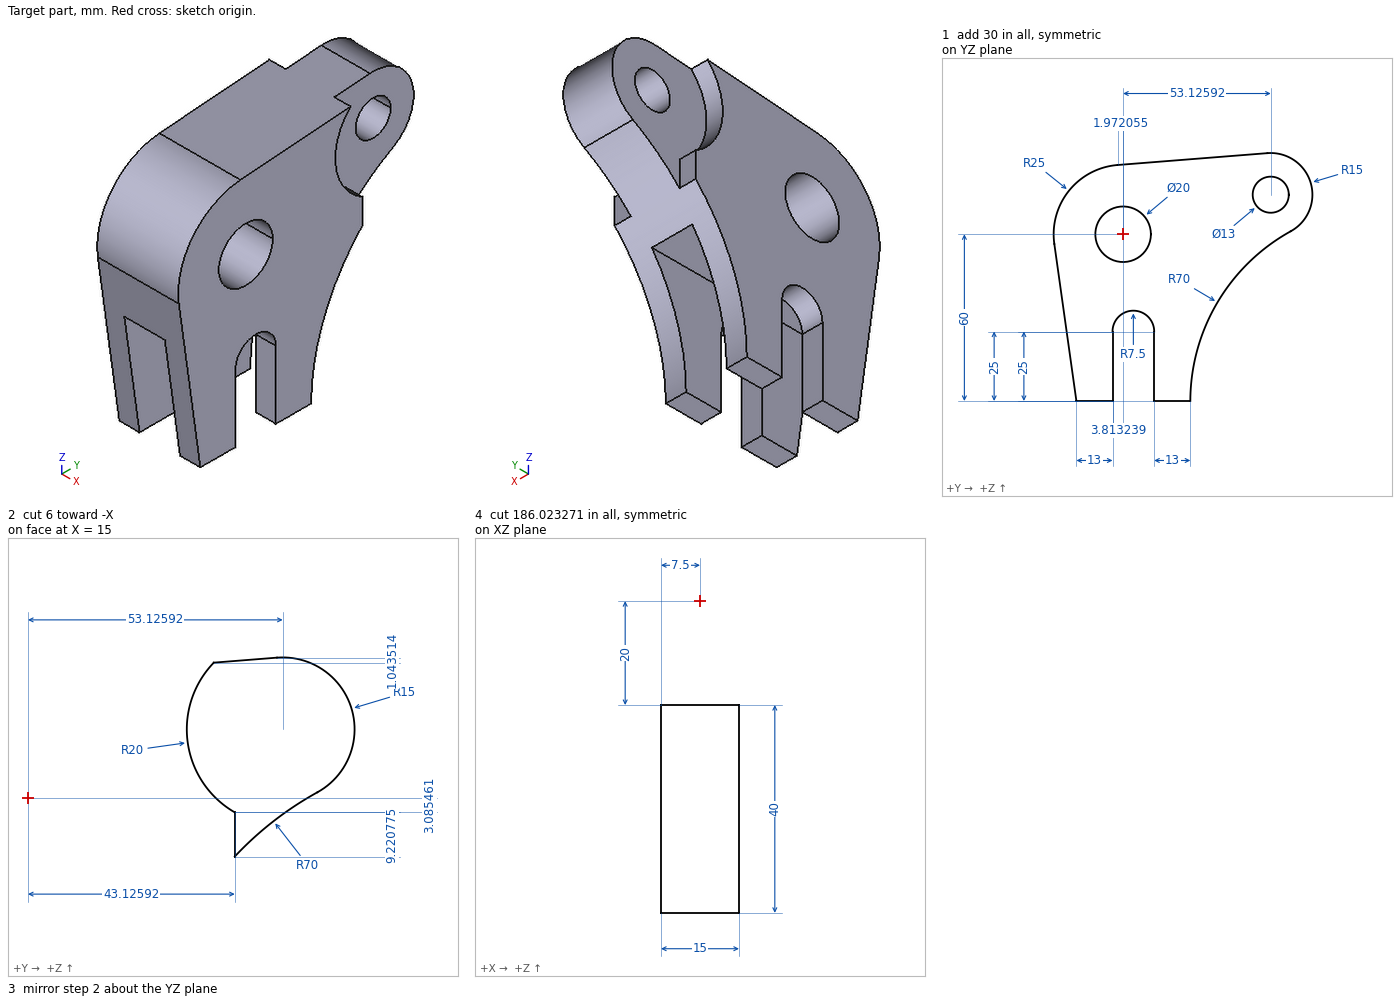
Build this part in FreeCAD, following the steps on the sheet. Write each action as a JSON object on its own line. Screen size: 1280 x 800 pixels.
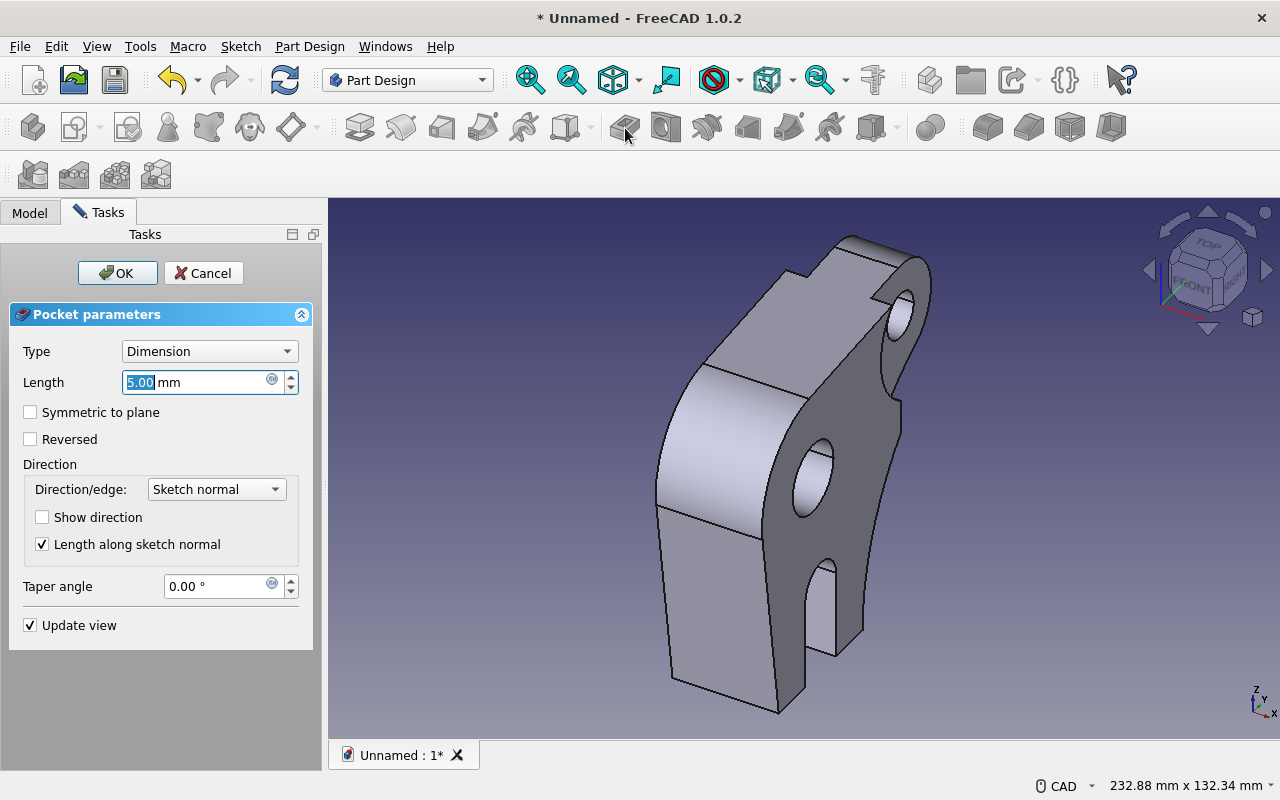
{"action": "type", "text": "186.023271"}
{"action": "key", "text": "Tab"}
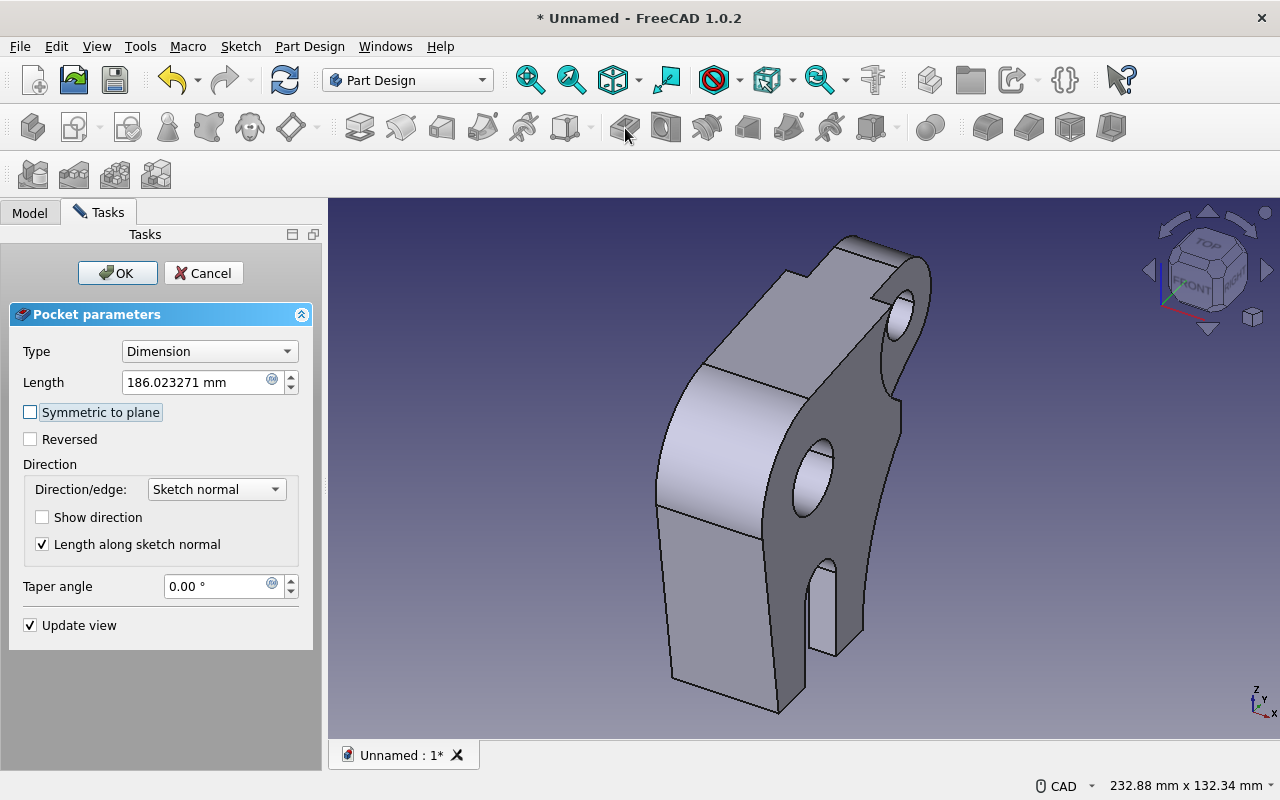
{"action": "left_click", "coordinate": [31, 412]}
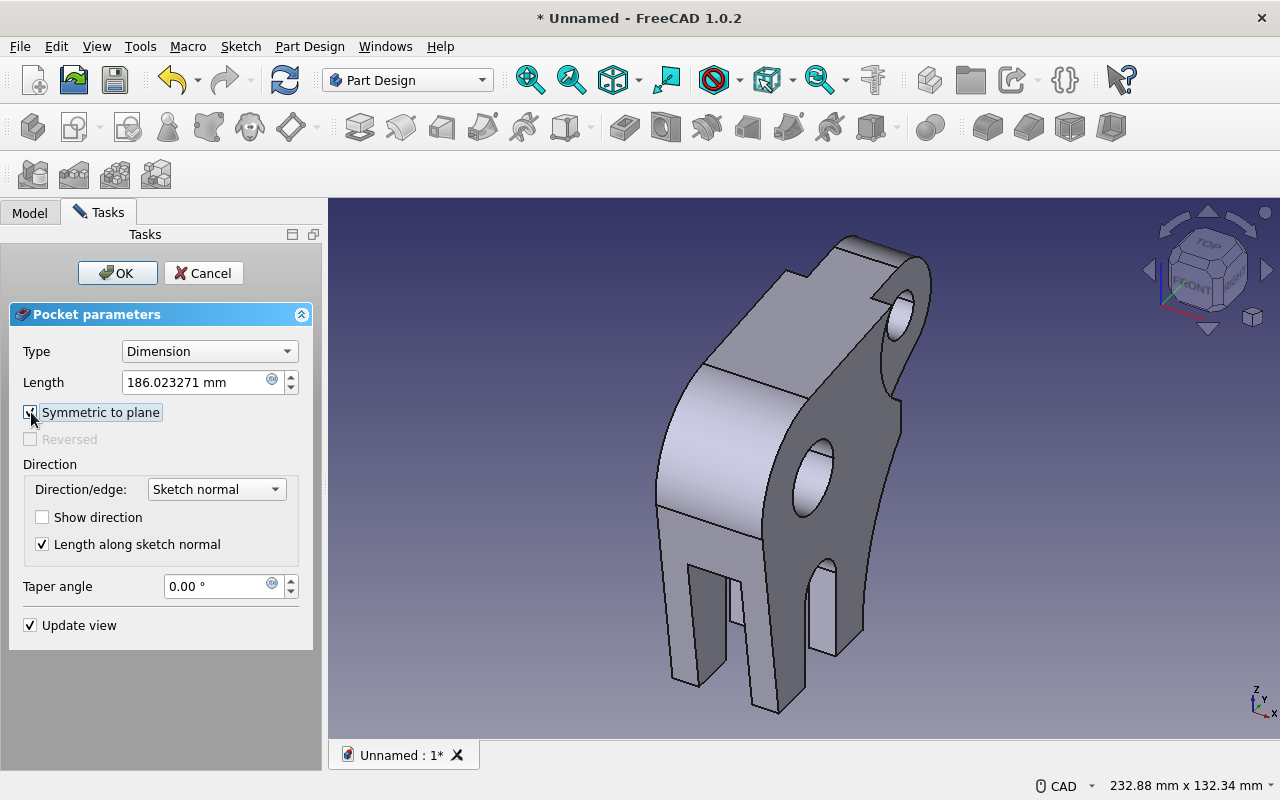
{"action": "left_click", "coordinate": [118, 273]}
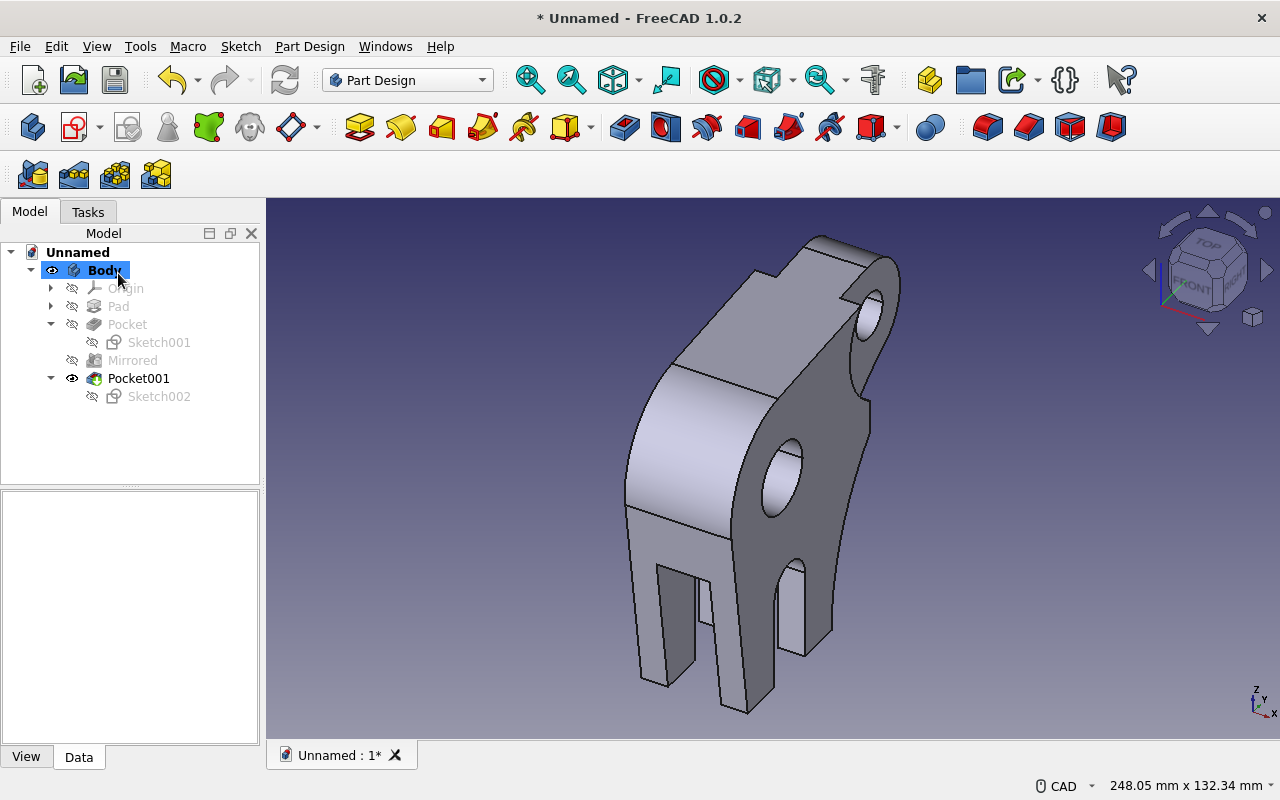
{"action": "key", "text": "0"}